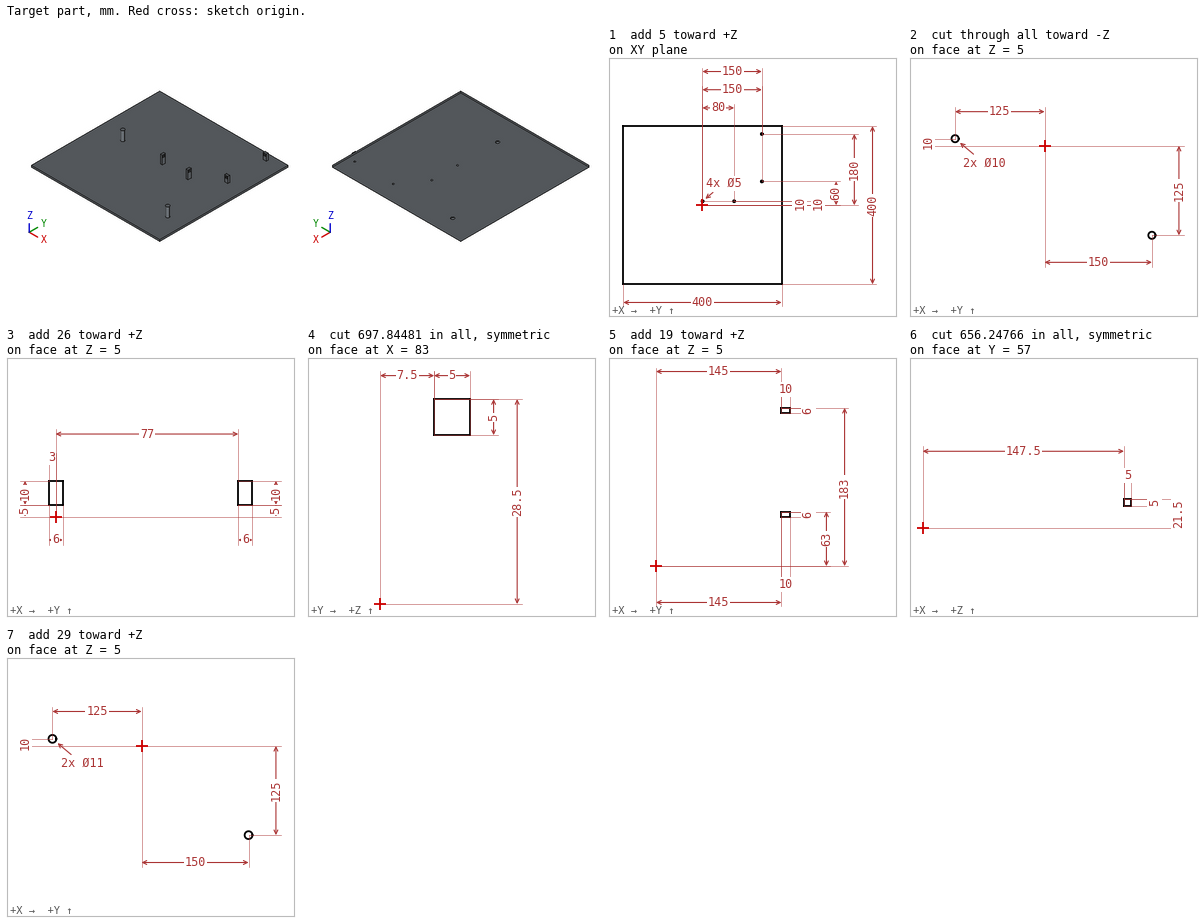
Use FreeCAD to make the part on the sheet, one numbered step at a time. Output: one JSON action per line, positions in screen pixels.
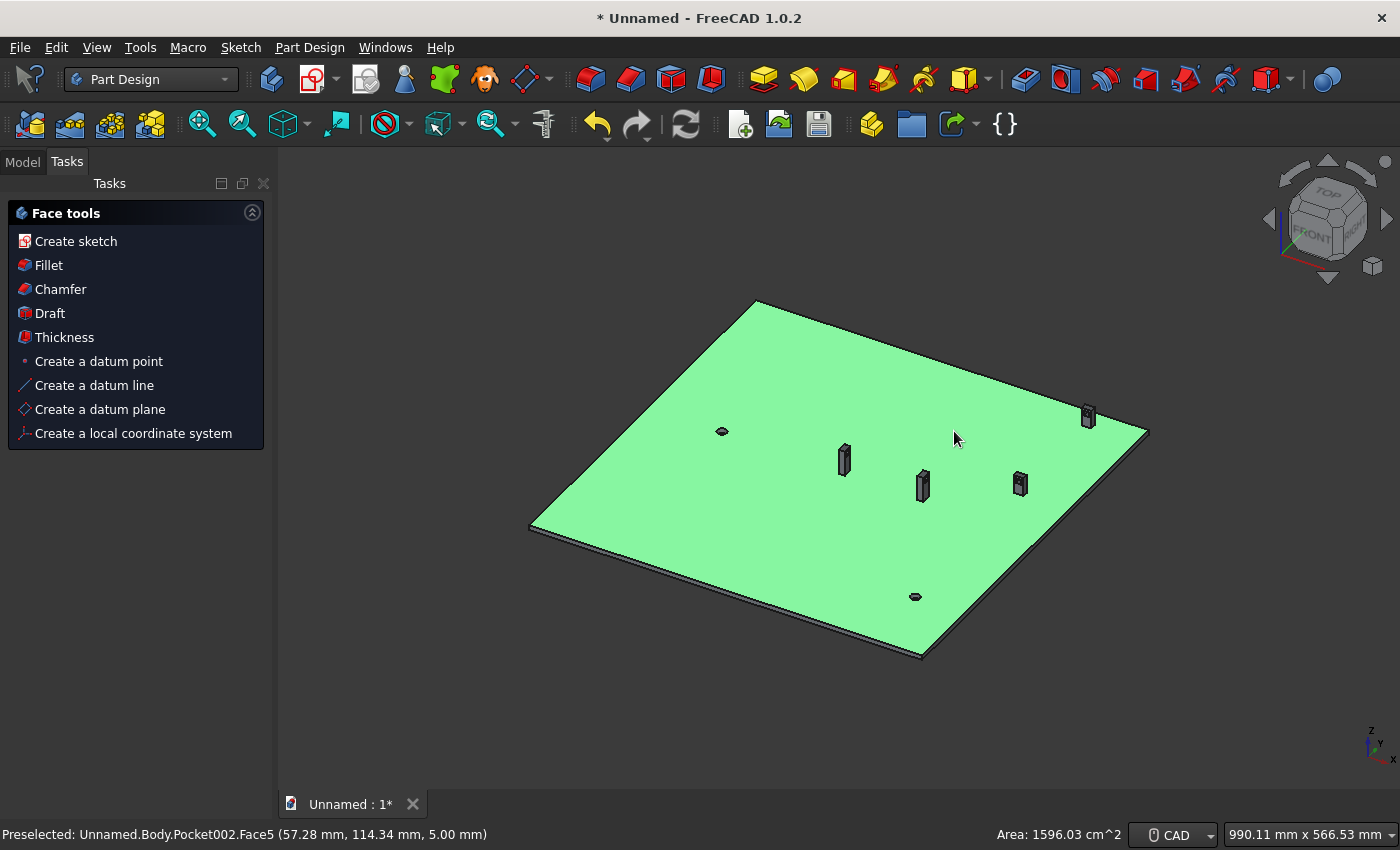
{"action": "left_click", "coordinate": [312, 80]}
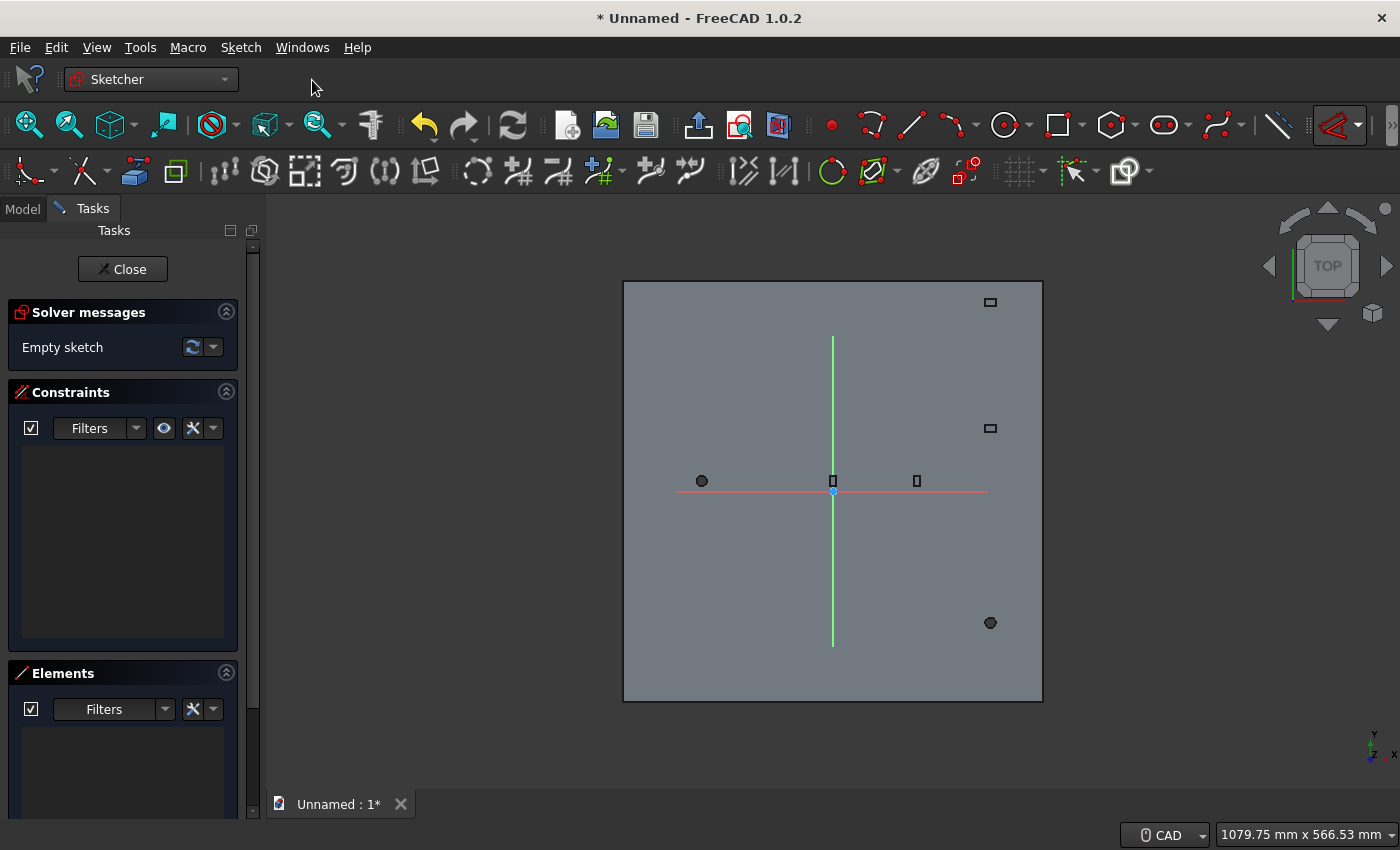
{"action": "scroll", "coordinate": [913, 601], "scroll_direction": "up", "scroll_amount": 4}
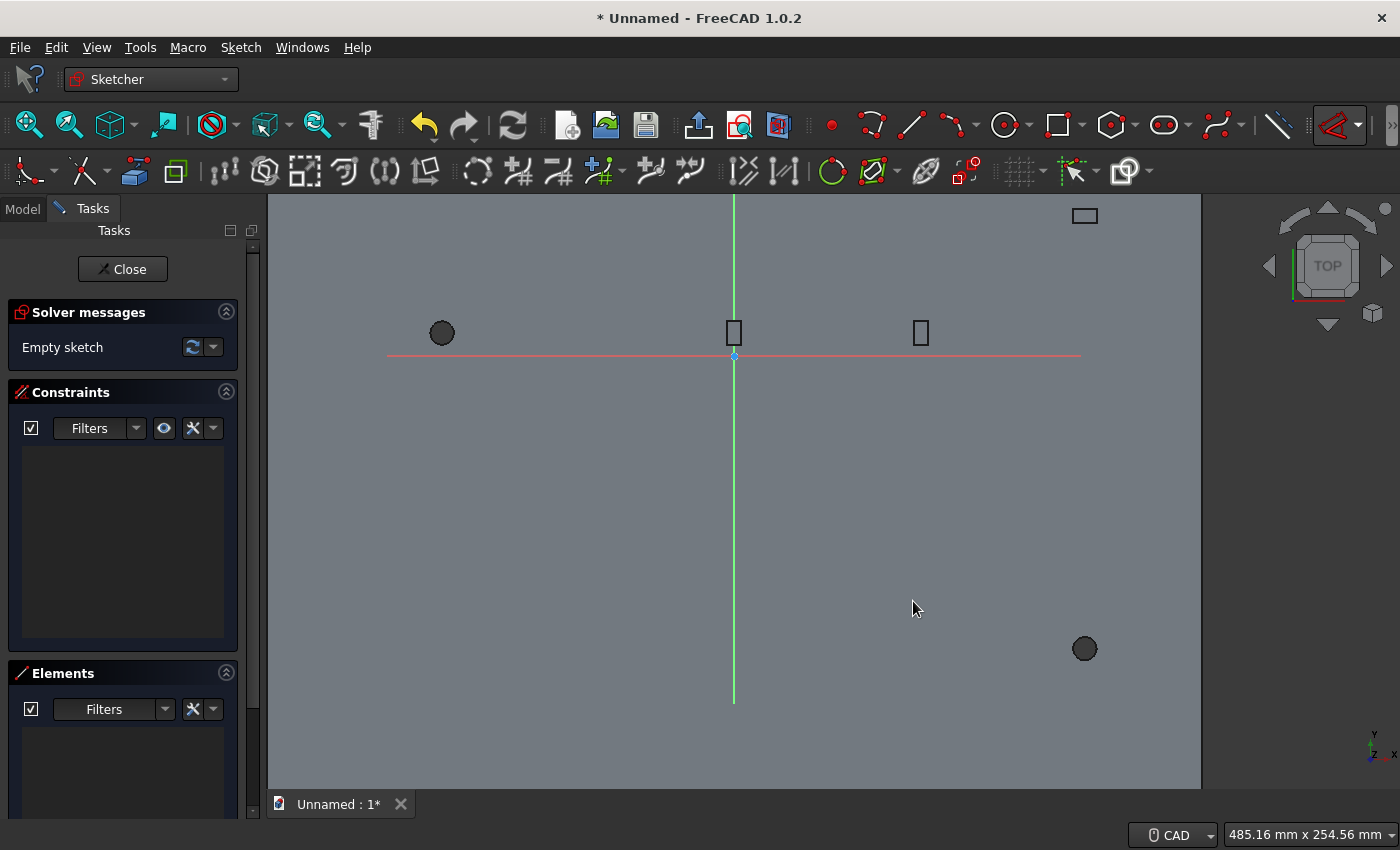
{"action": "key", "text": "g c"}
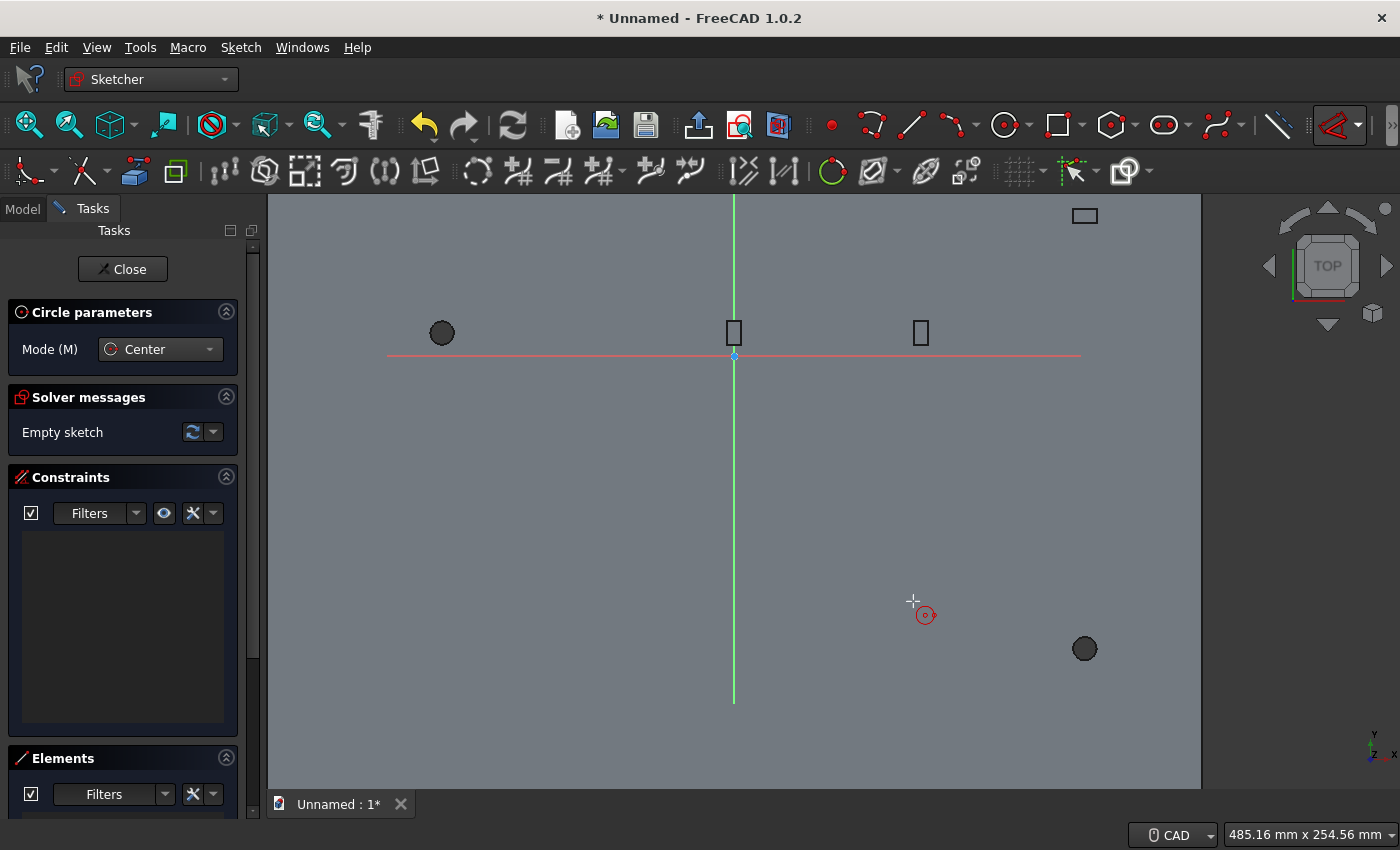
{"action": "scroll", "coordinate": [442, 333], "scroll_direction": "up", "scroll_amount": 3}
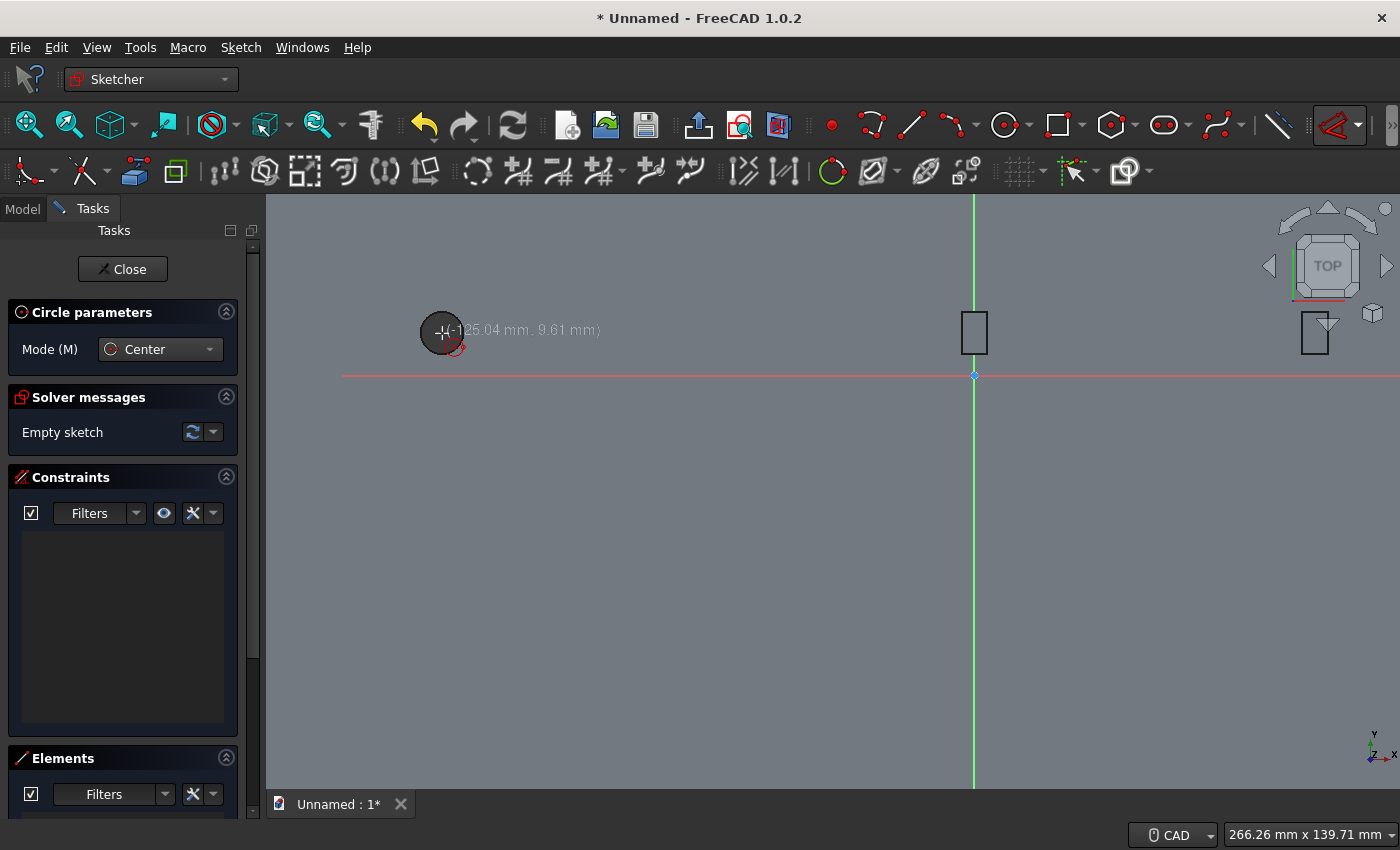
{"action": "left_click", "coordinate": [442, 333]}
{"action": "left_click", "coordinate": [459, 316]}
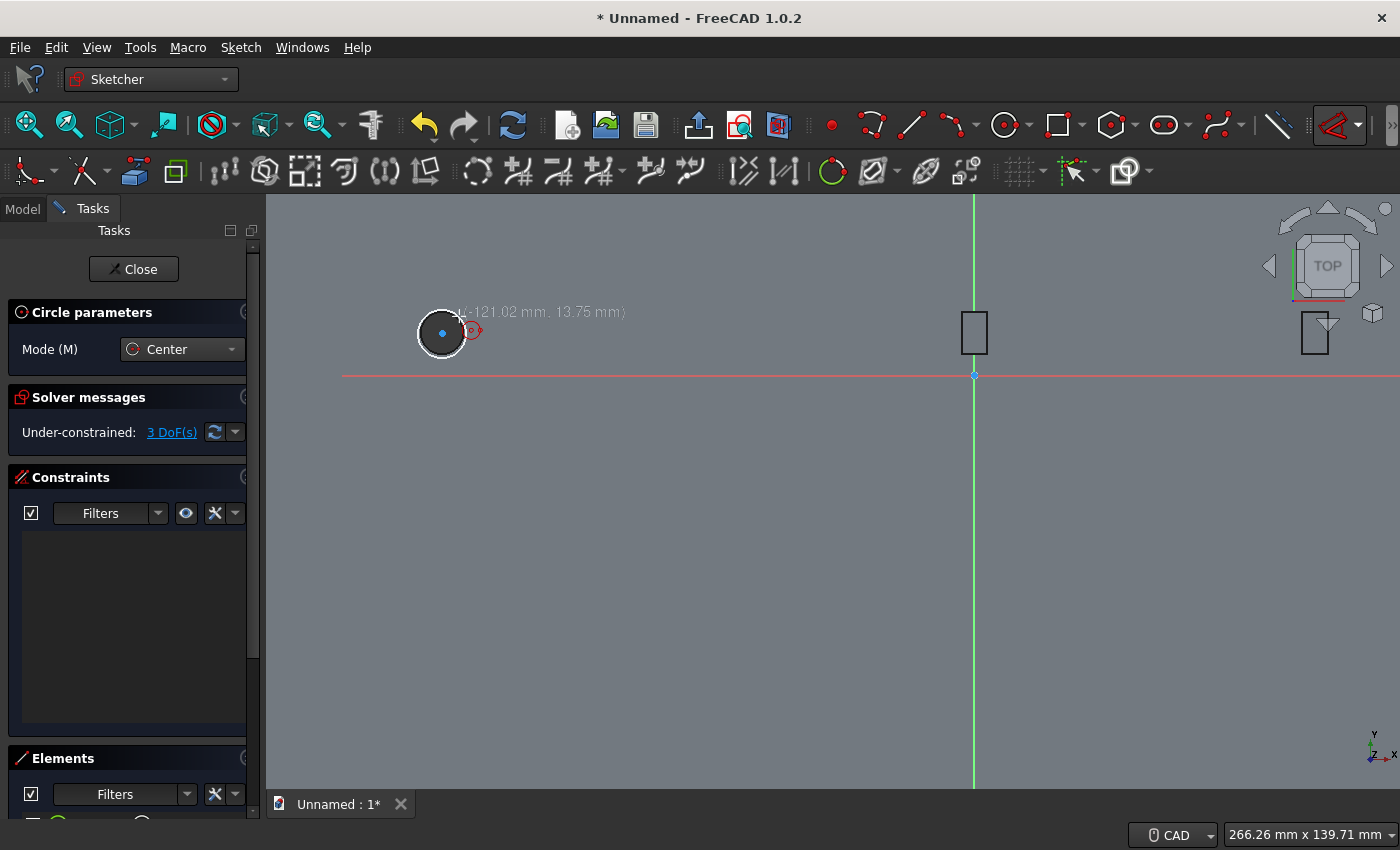
{"action": "scroll", "coordinate": [444, 335], "scroll_direction": "down", "scroll_amount": 3}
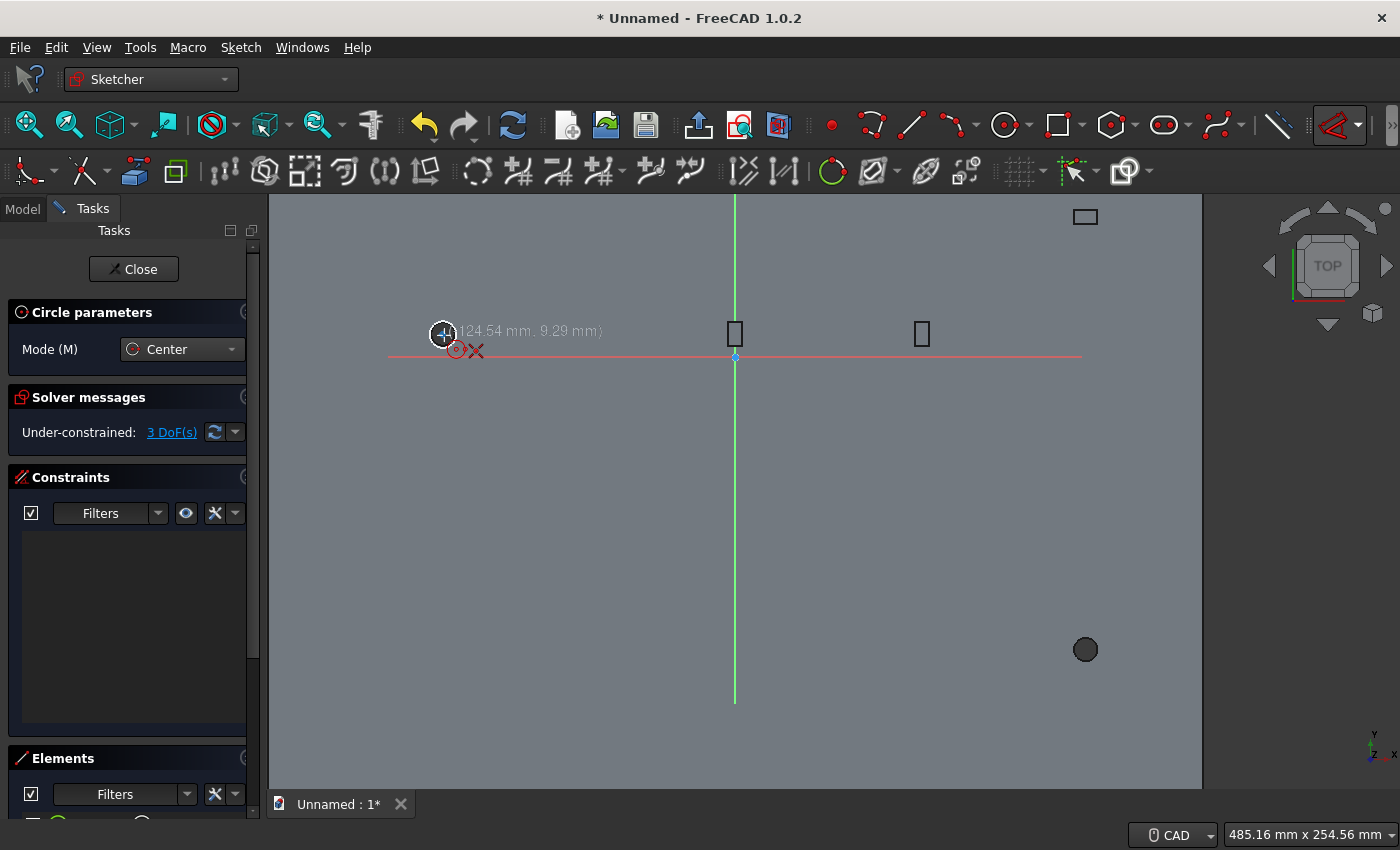
{"action": "scroll", "coordinate": [1086, 650], "scroll_direction": "up", "scroll_amount": 3}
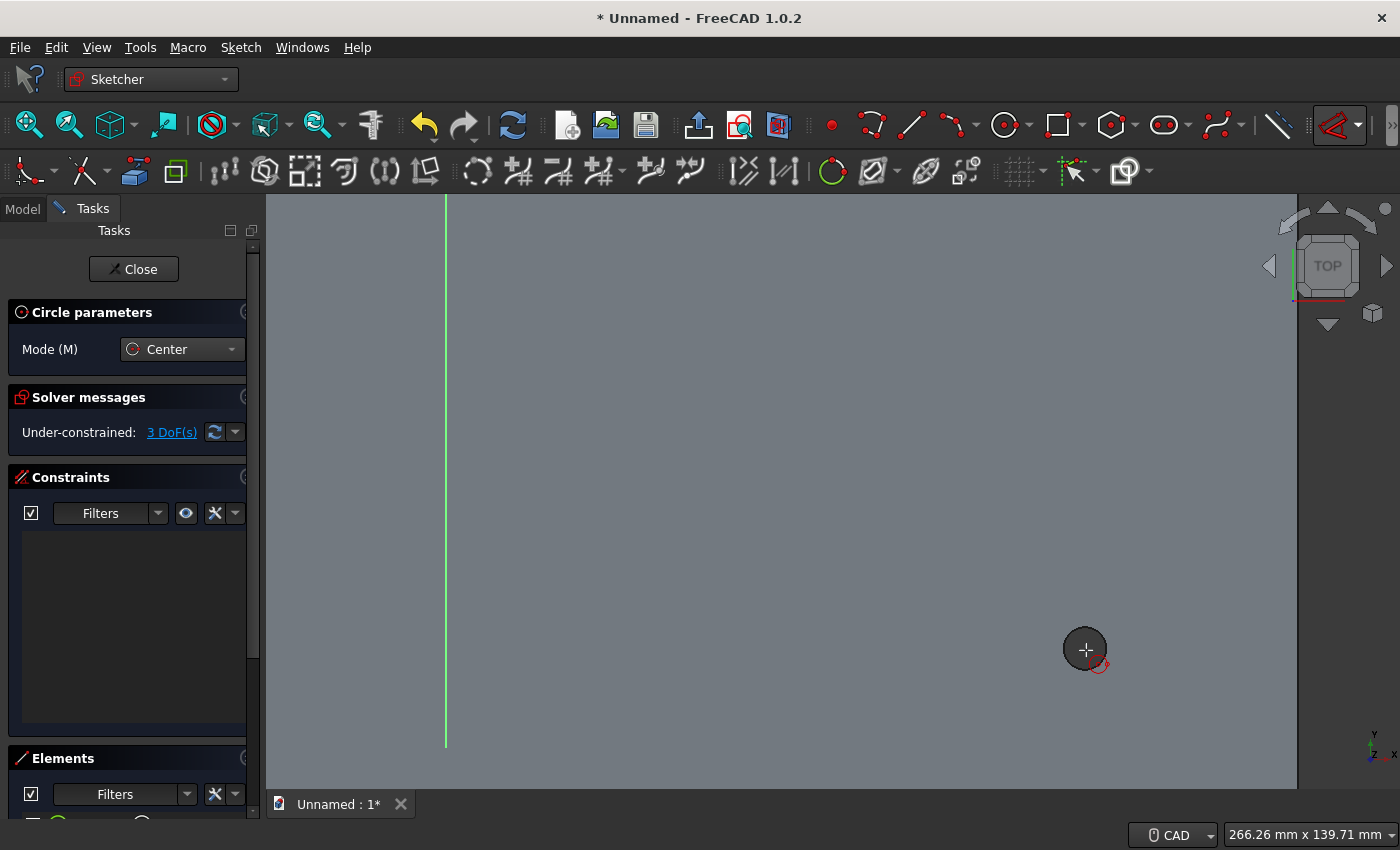
{"action": "left_click", "coordinate": [1085, 649]}
{"action": "left_click", "coordinate": [1102, 632]}
{"action": "key", "text": "Escape"}